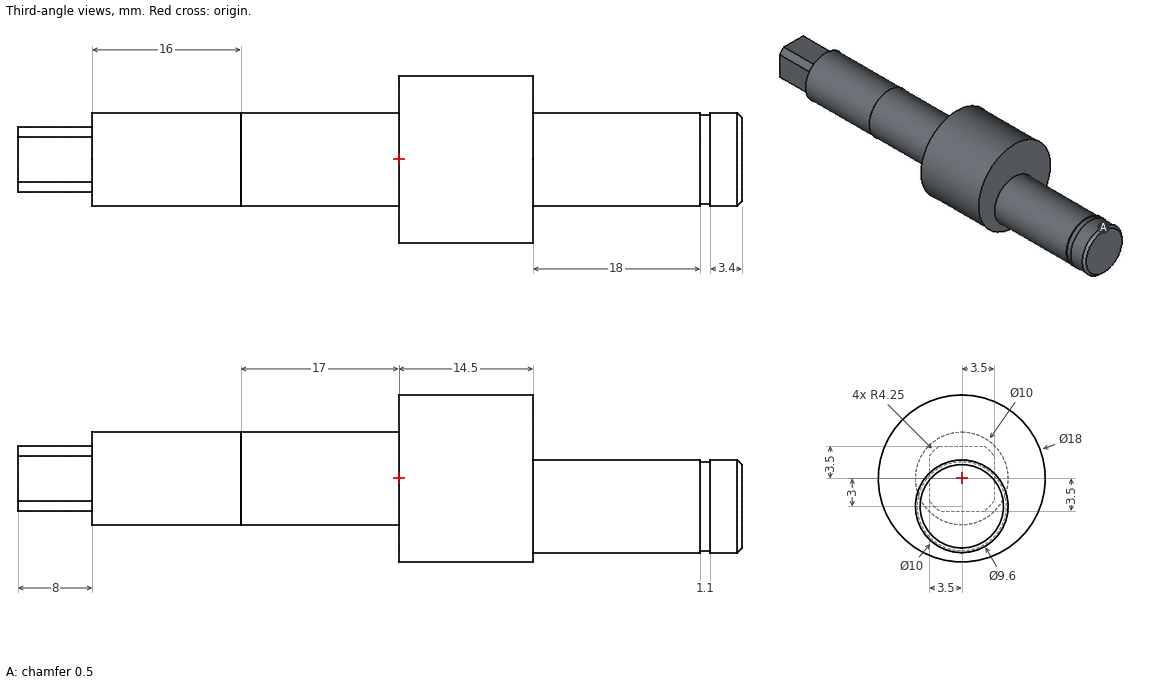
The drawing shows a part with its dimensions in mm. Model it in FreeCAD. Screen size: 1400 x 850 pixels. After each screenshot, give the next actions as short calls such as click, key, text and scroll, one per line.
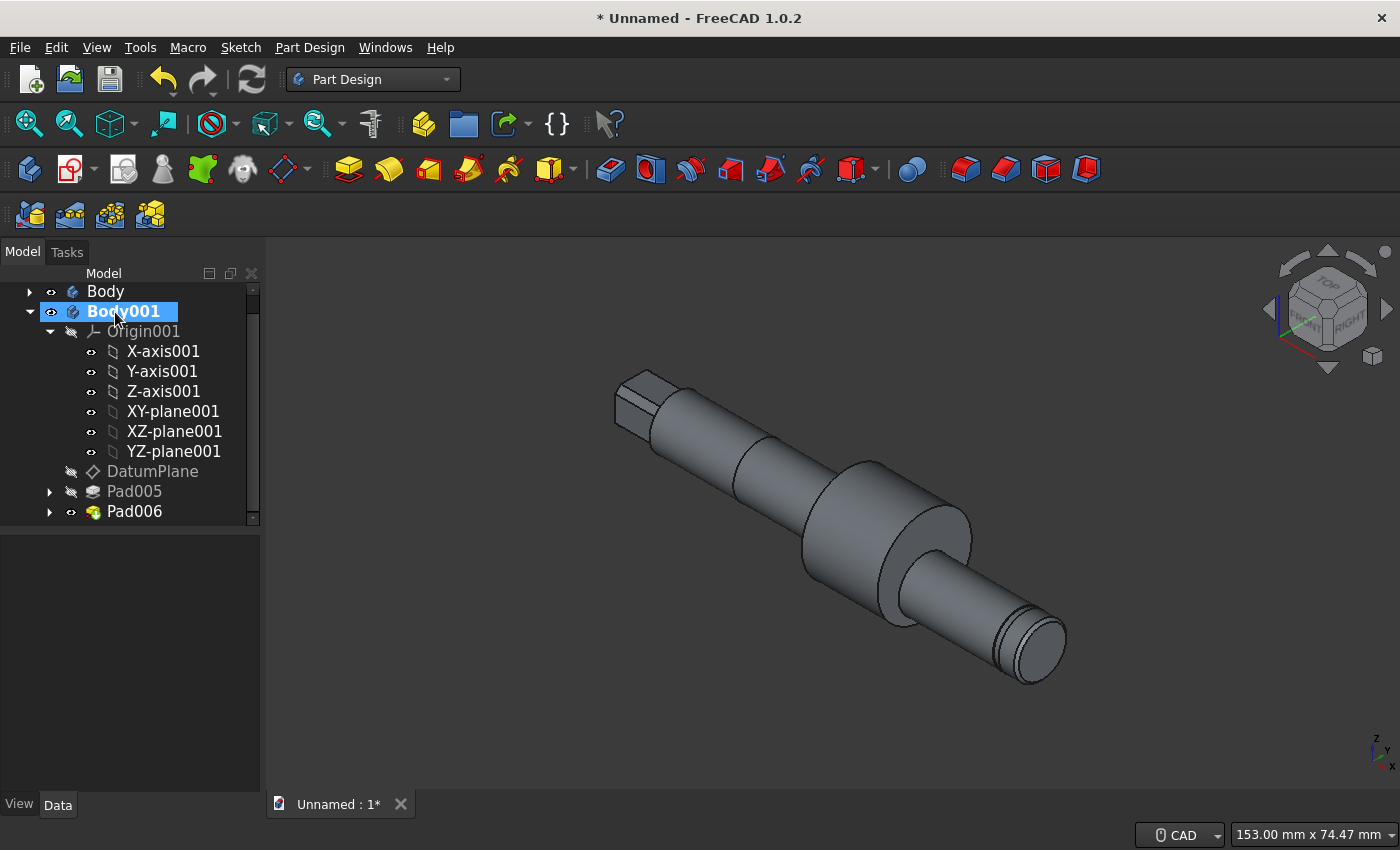
click(30, 124)